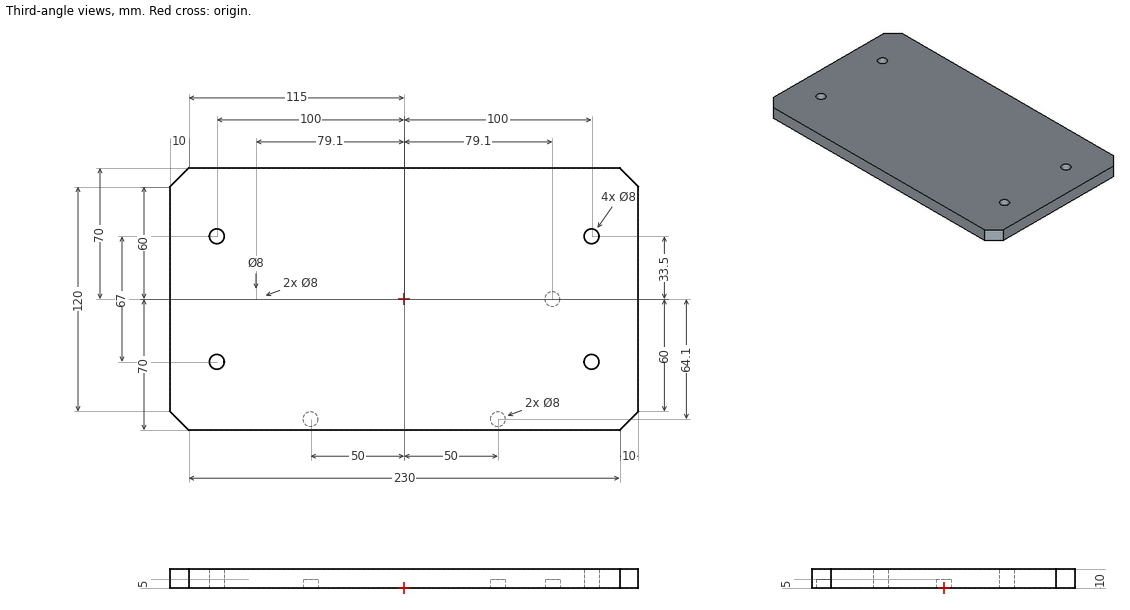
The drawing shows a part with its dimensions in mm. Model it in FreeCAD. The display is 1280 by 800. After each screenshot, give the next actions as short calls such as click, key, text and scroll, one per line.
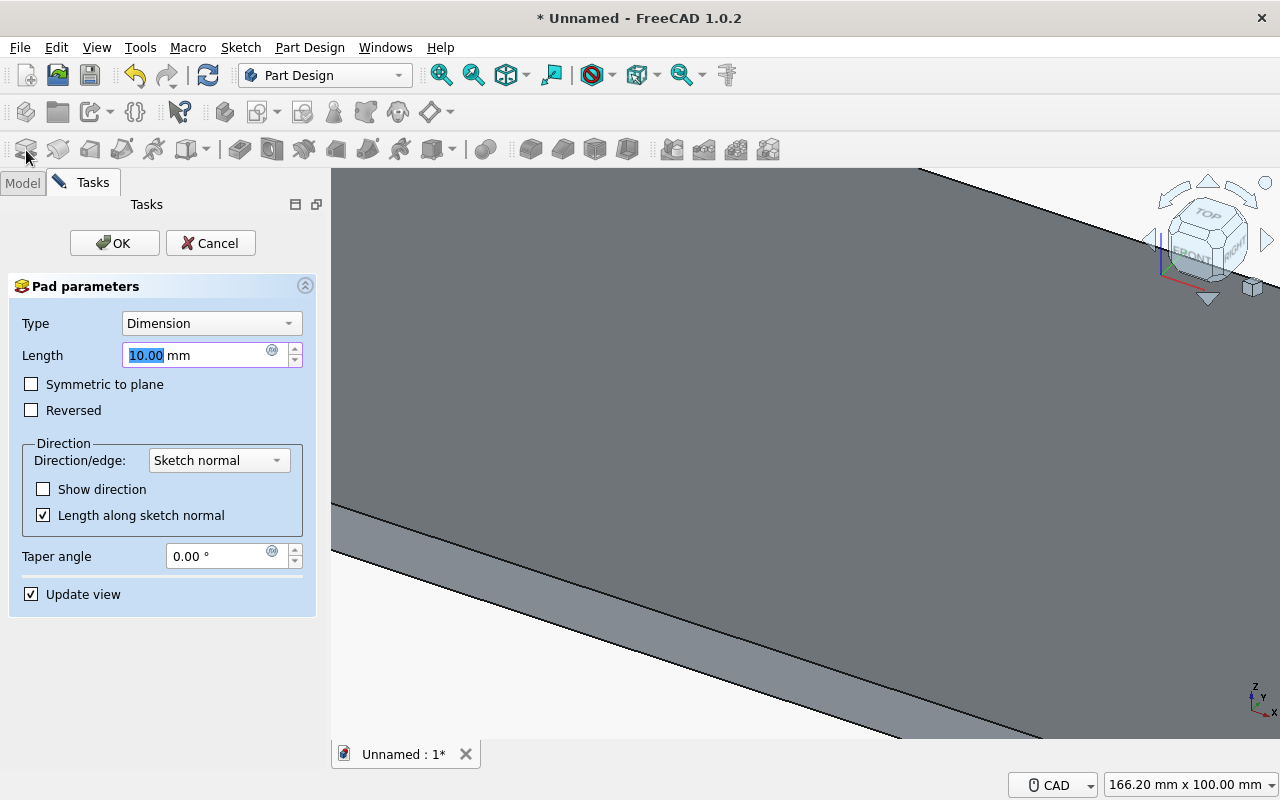
text(10)
key(Tab)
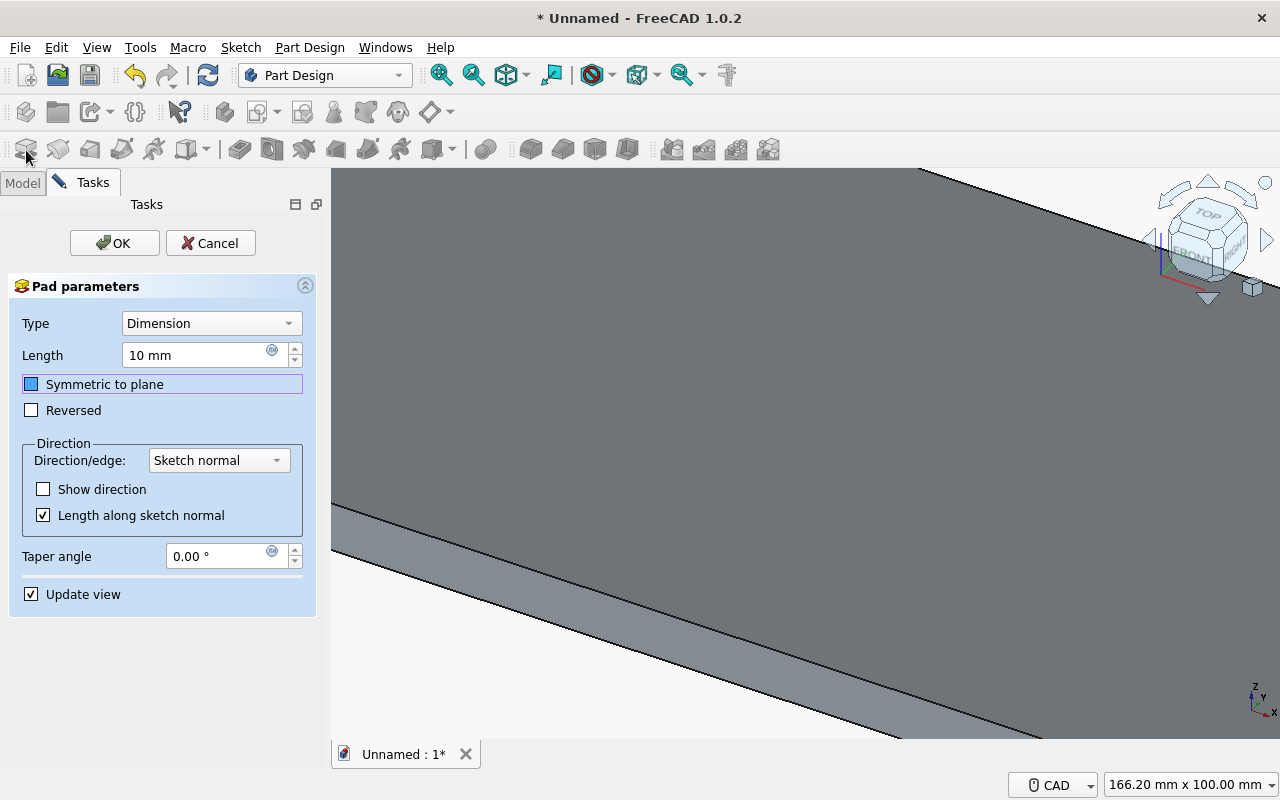
click(115, 243)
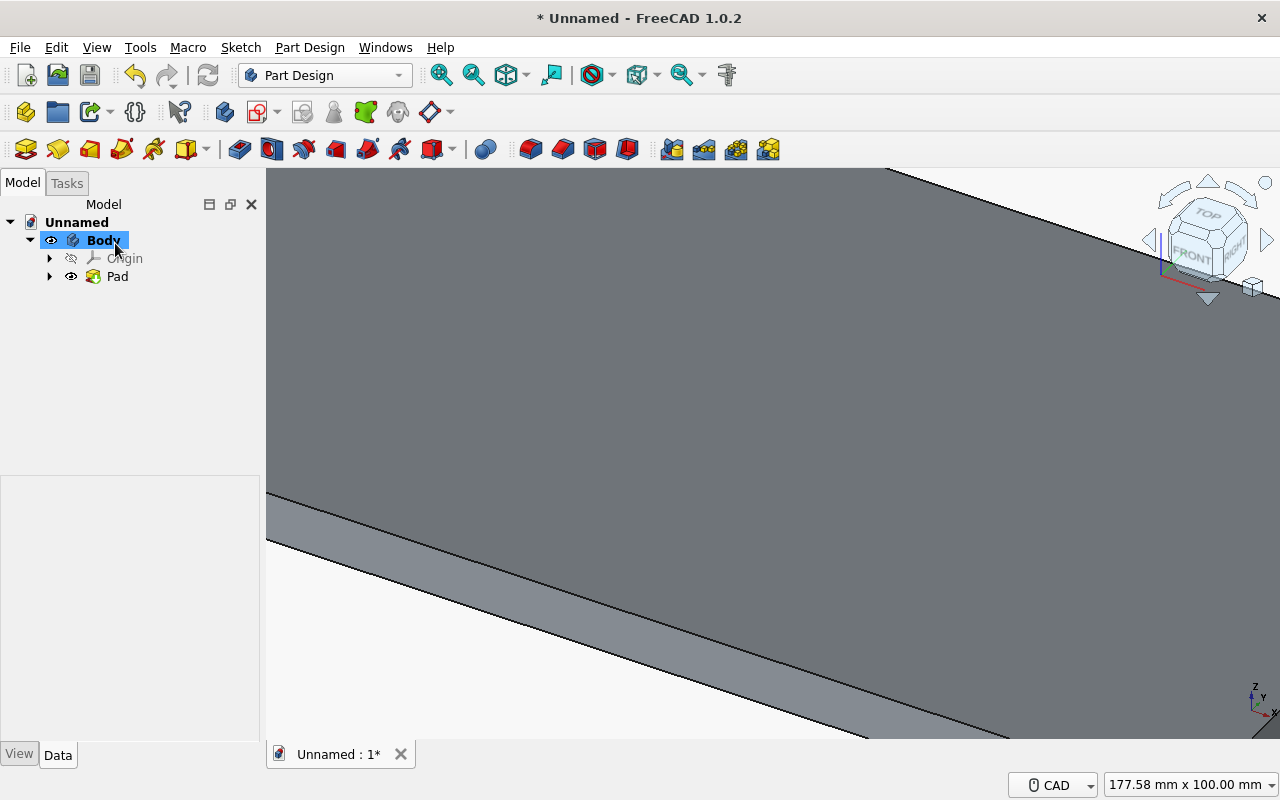
click(442, 76)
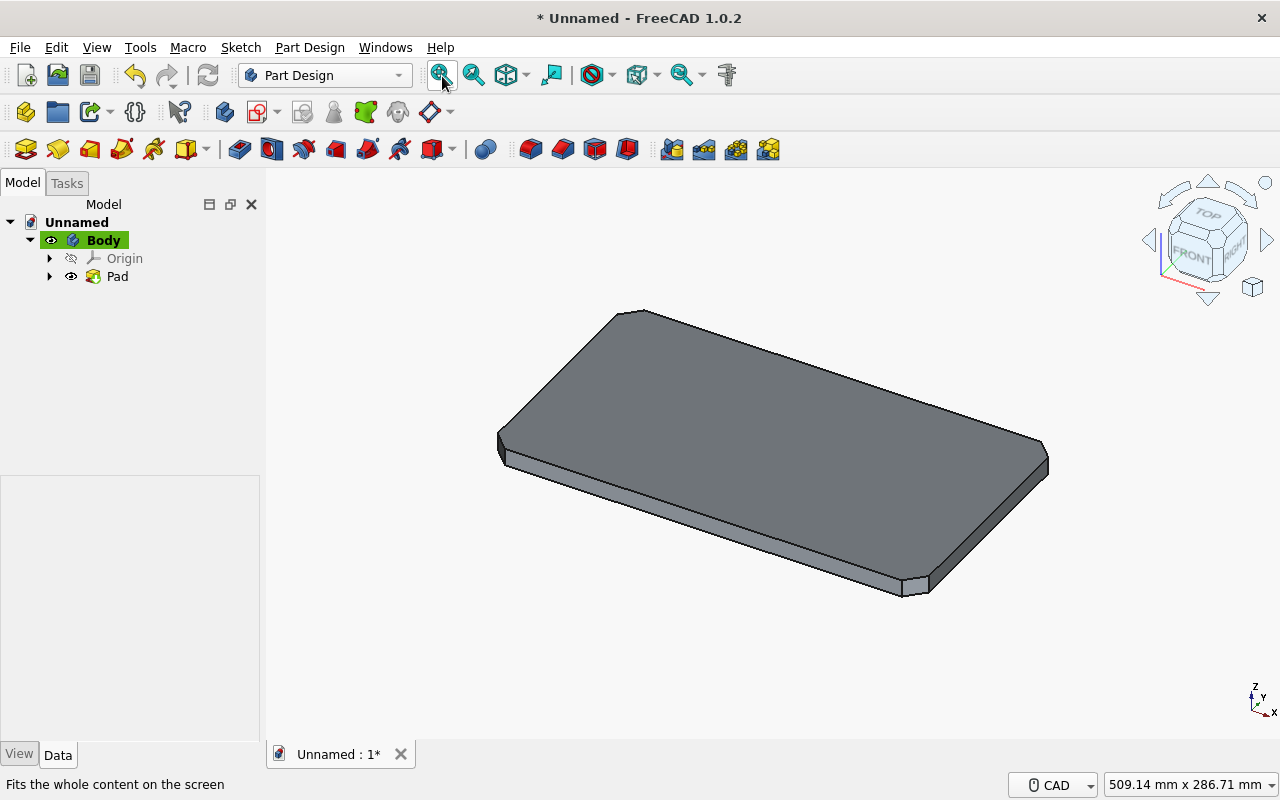
key(5)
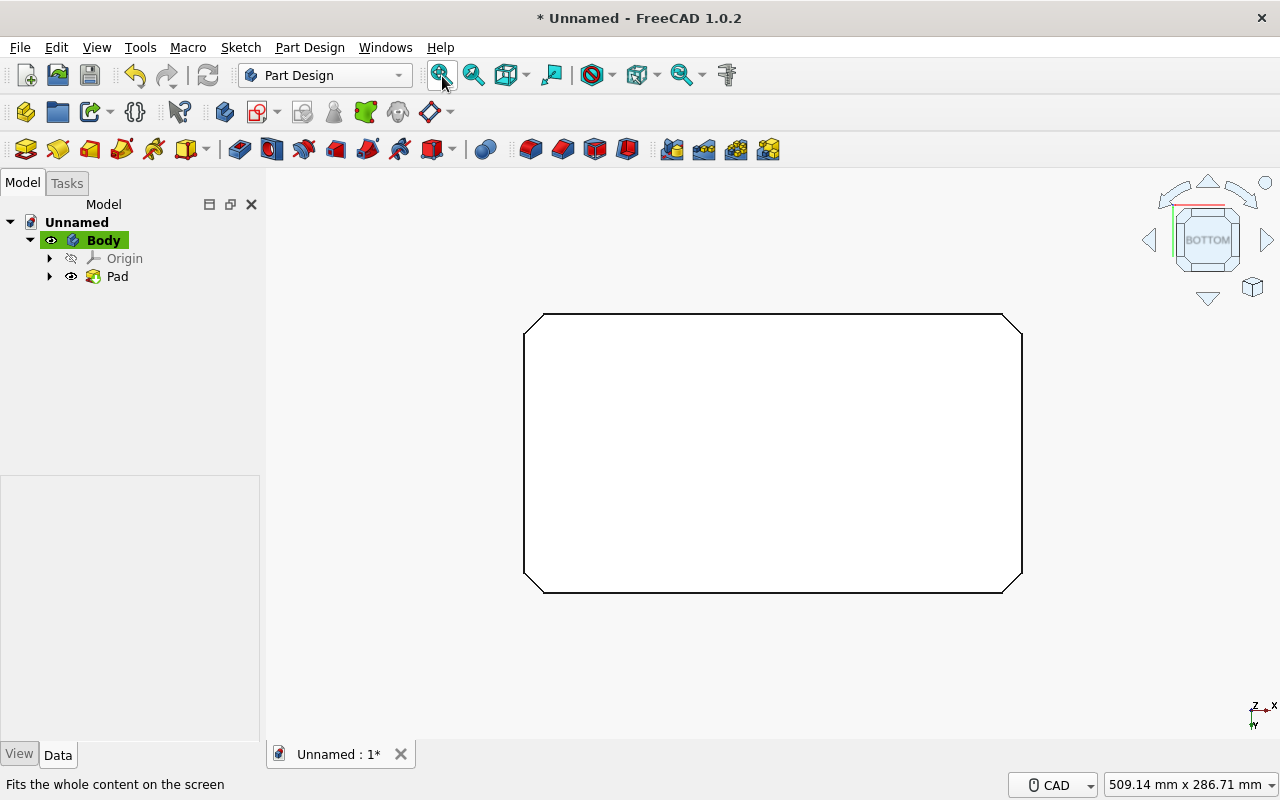
click(844, 452)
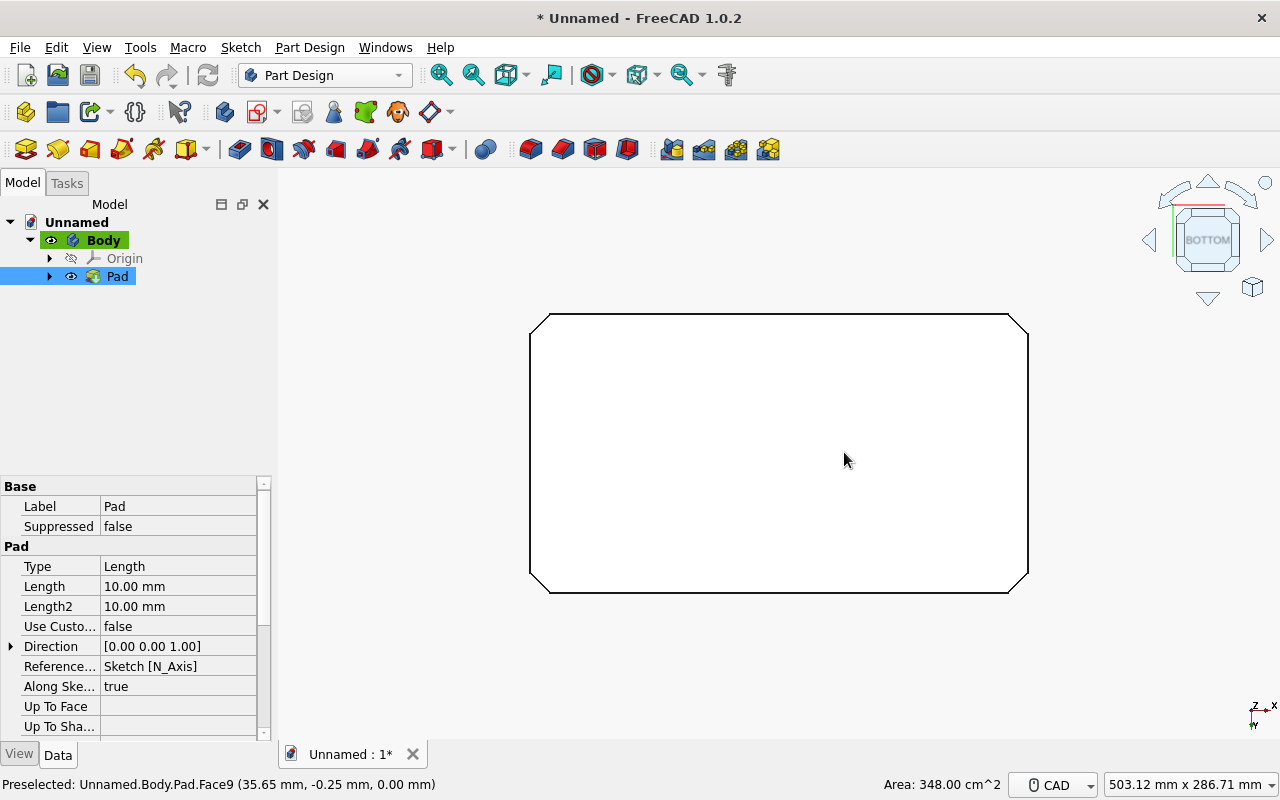
click(258, 112)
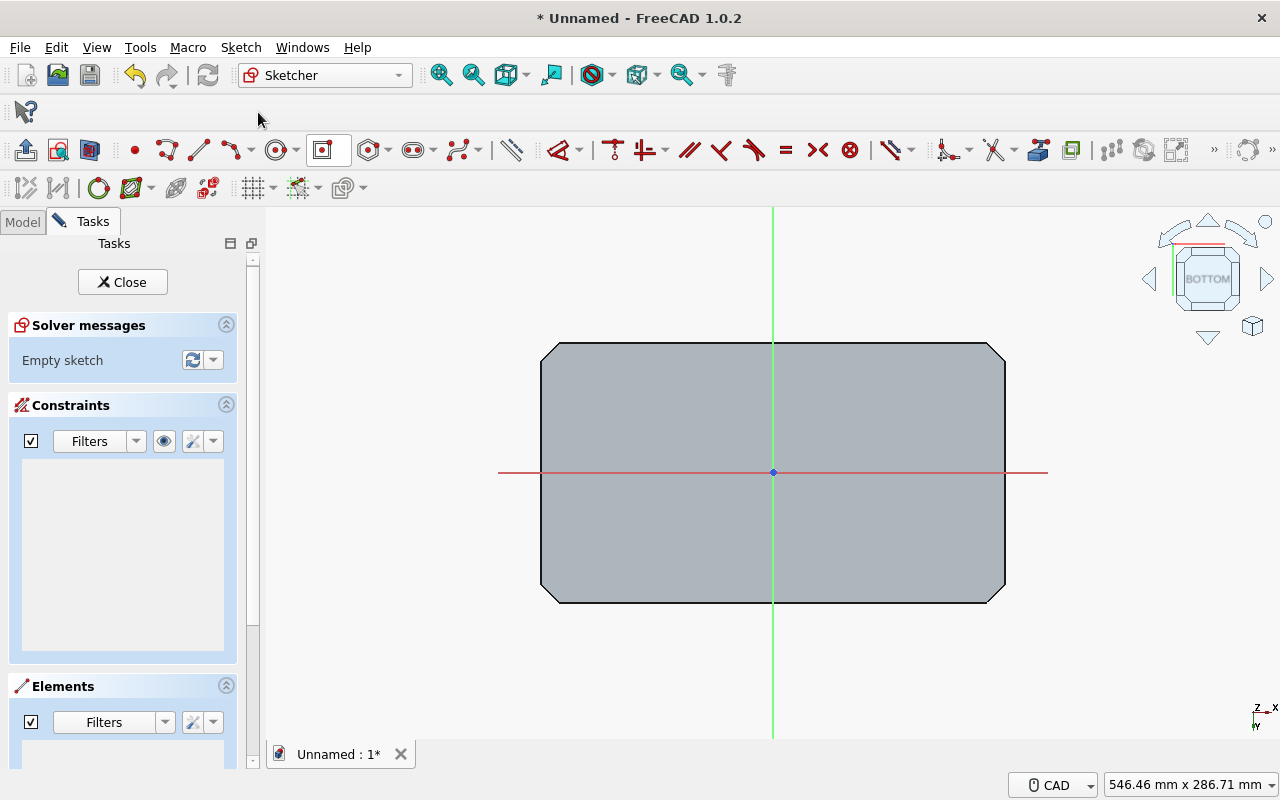
scroll(856, 473, up, 3)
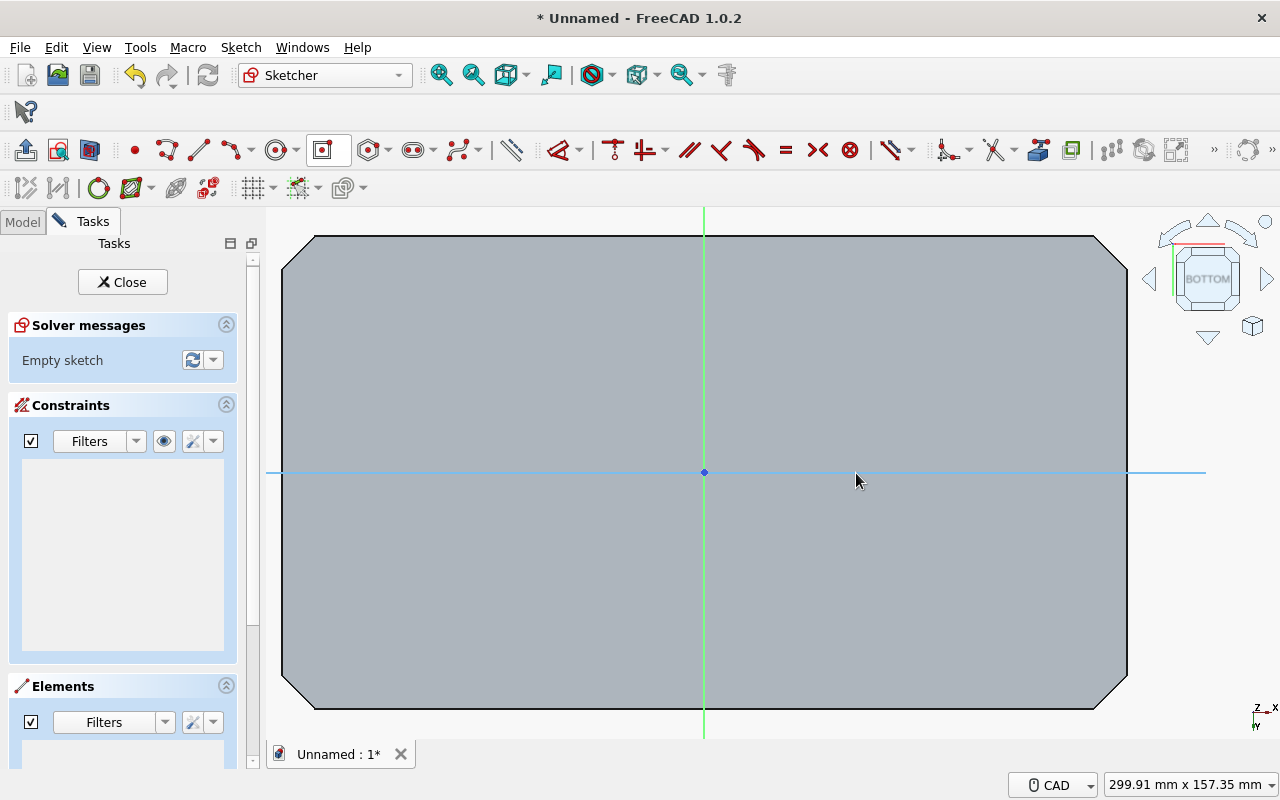
click(276, 150)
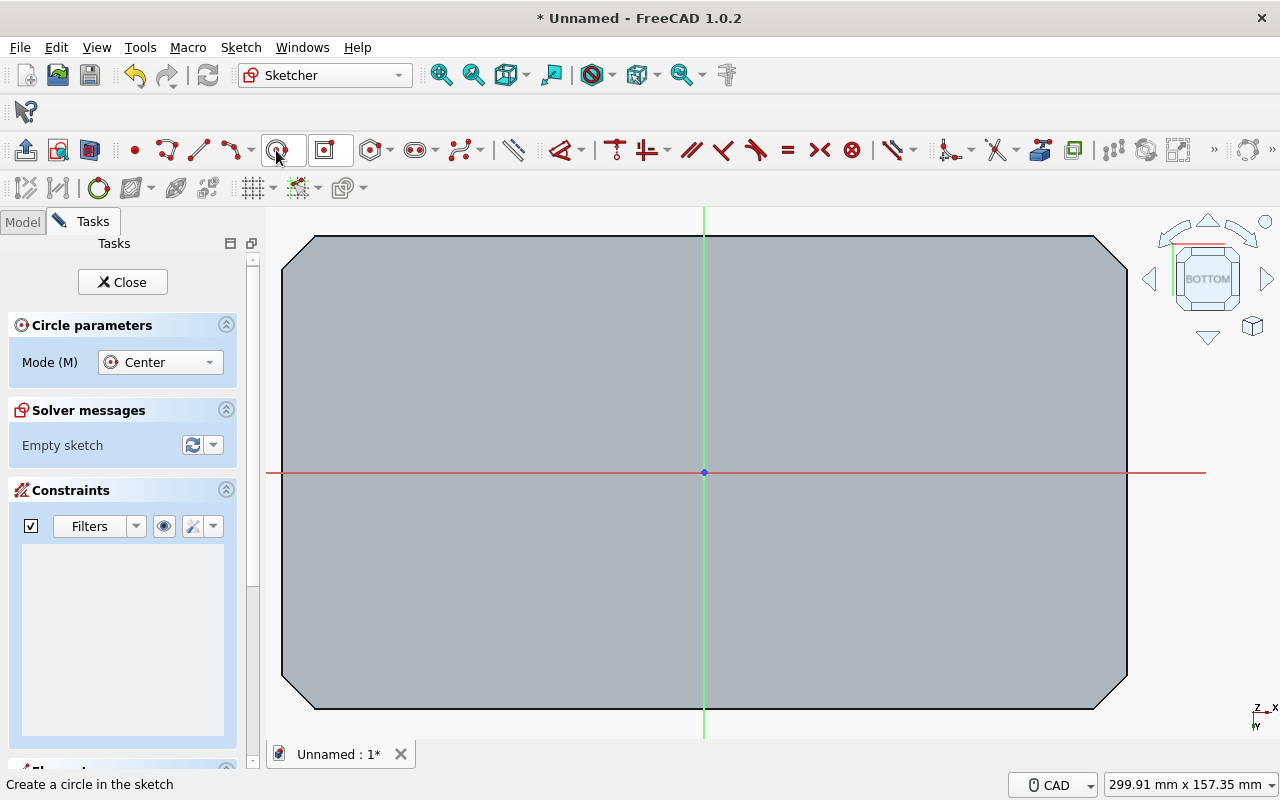
scroll(437, 473, up, 3)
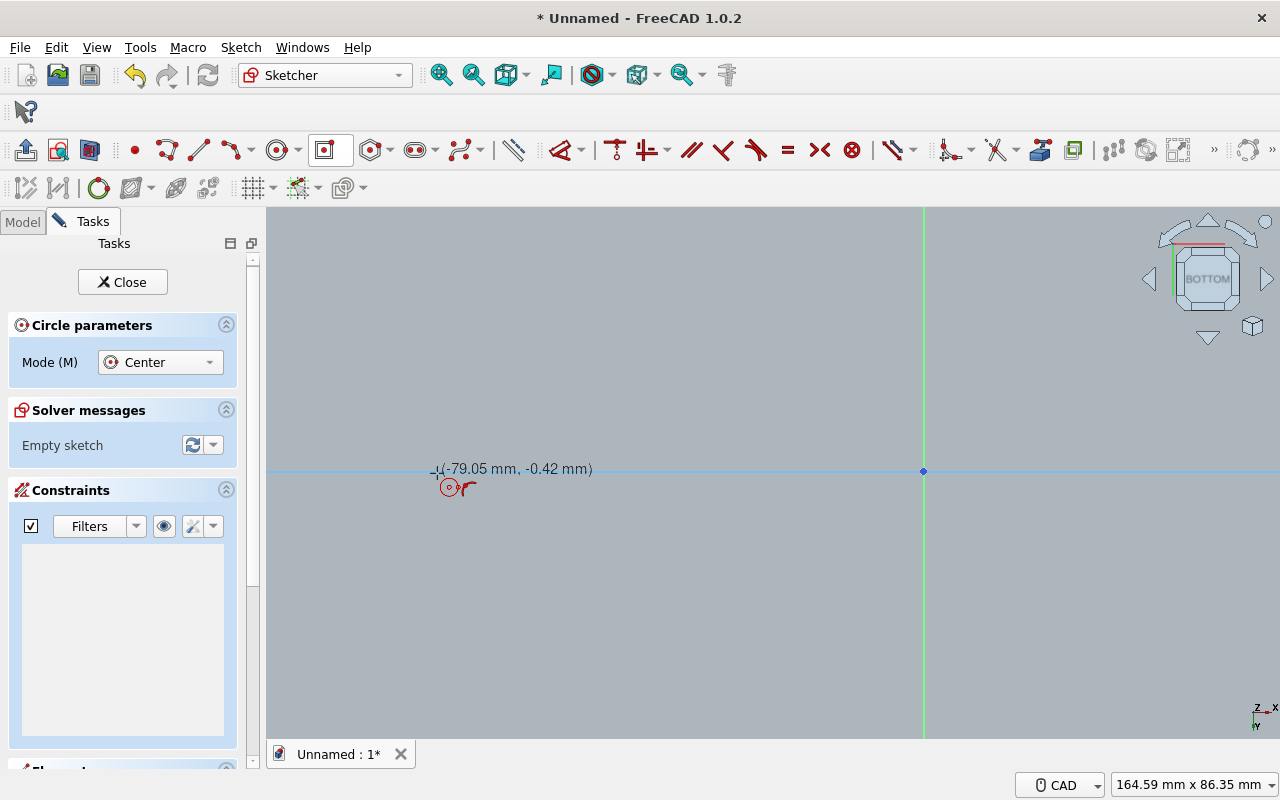
click(437, 472)
click(454, 454)